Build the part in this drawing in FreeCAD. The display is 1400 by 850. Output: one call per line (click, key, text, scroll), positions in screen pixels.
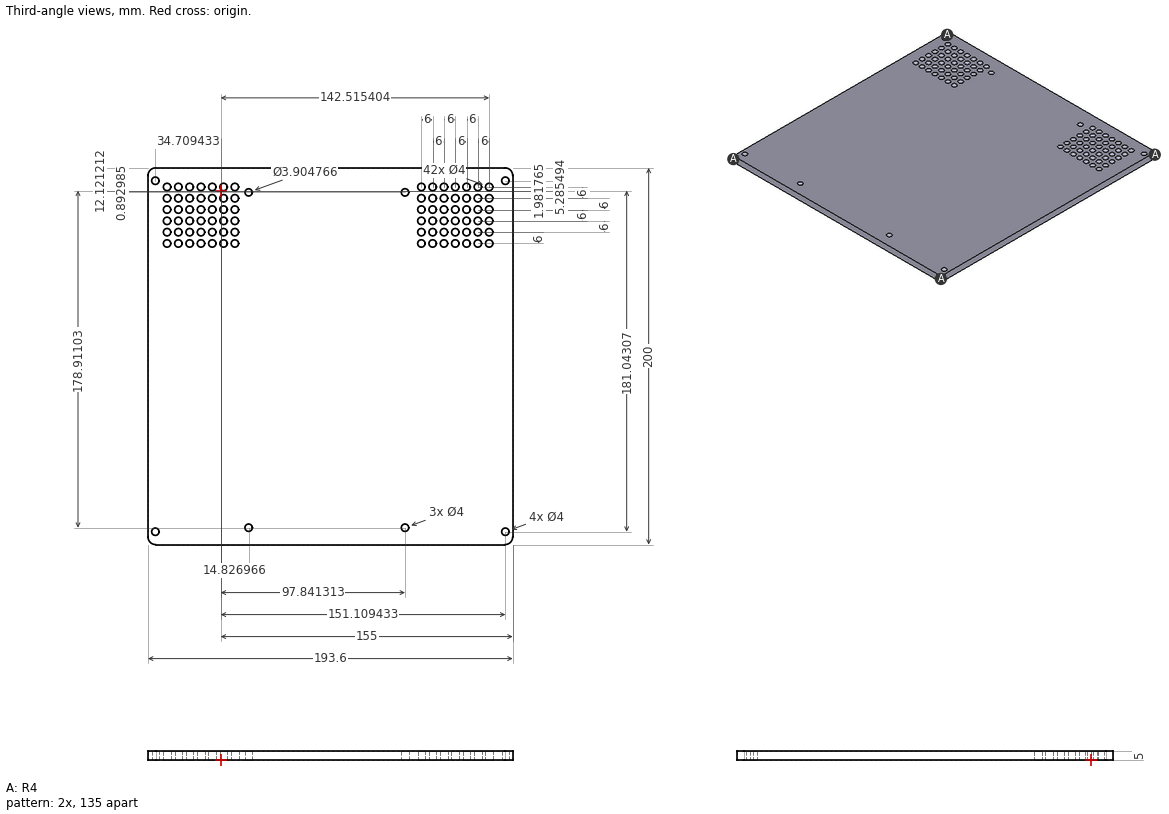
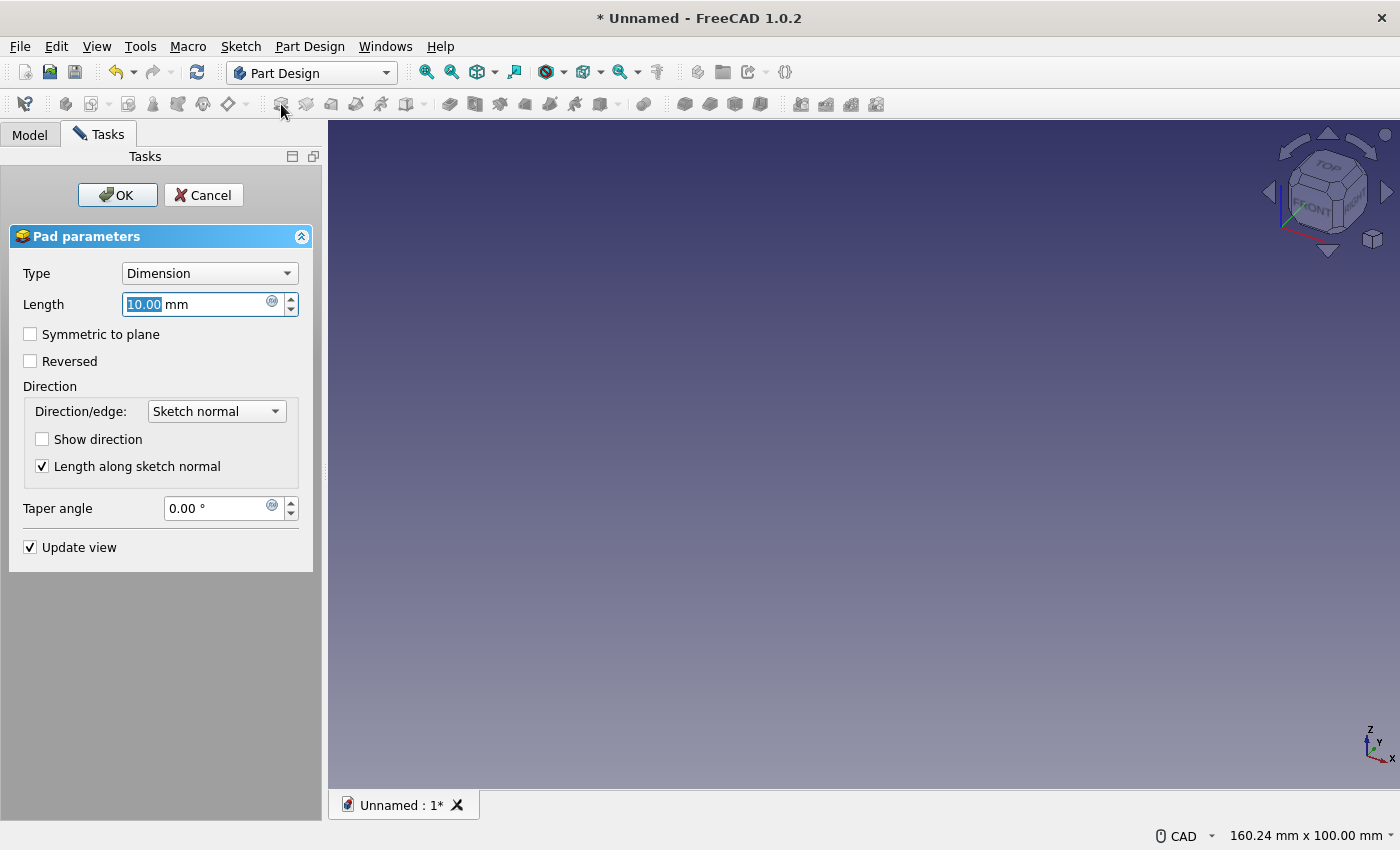
text(5)
key(Tab)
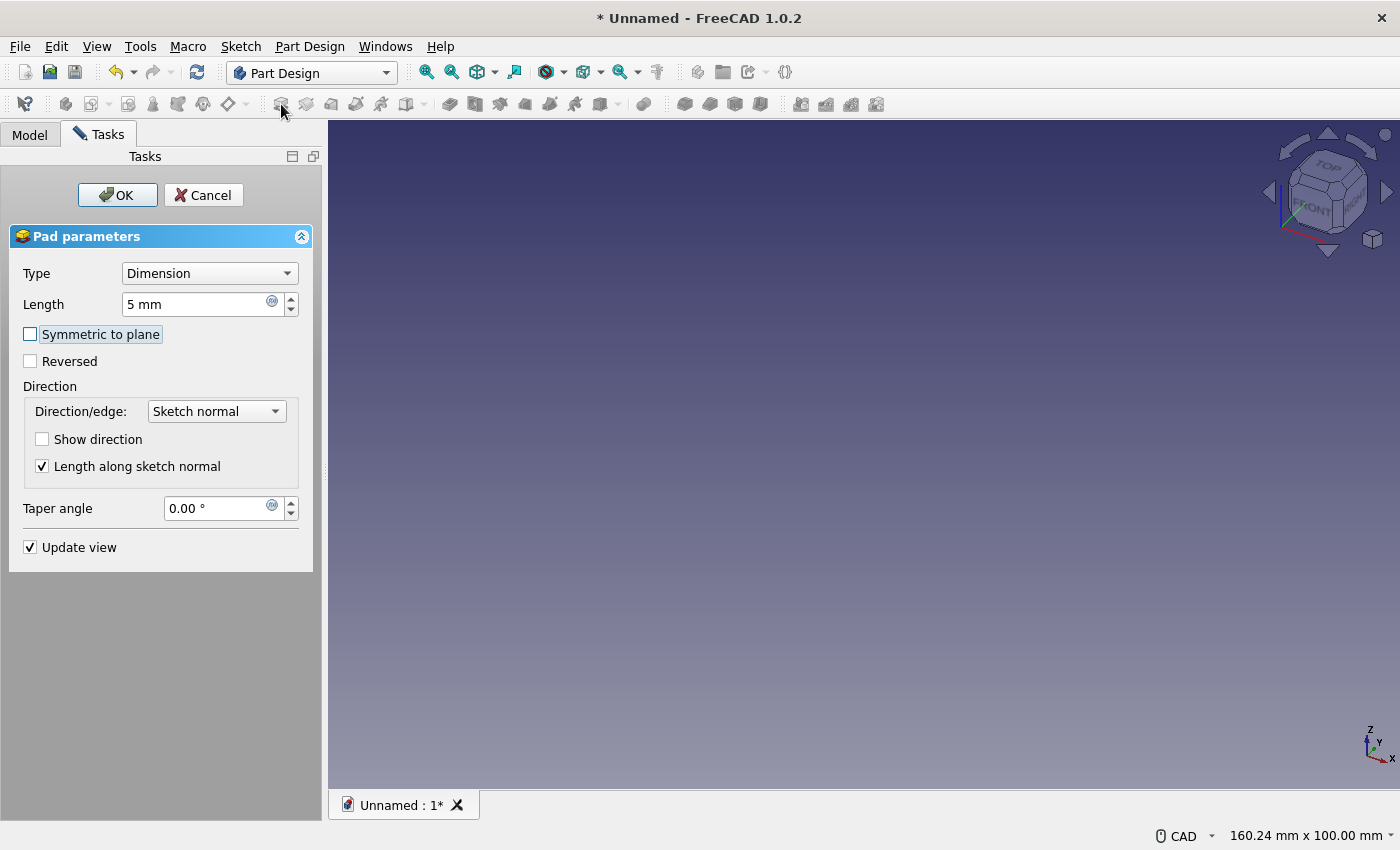
click(118, 195)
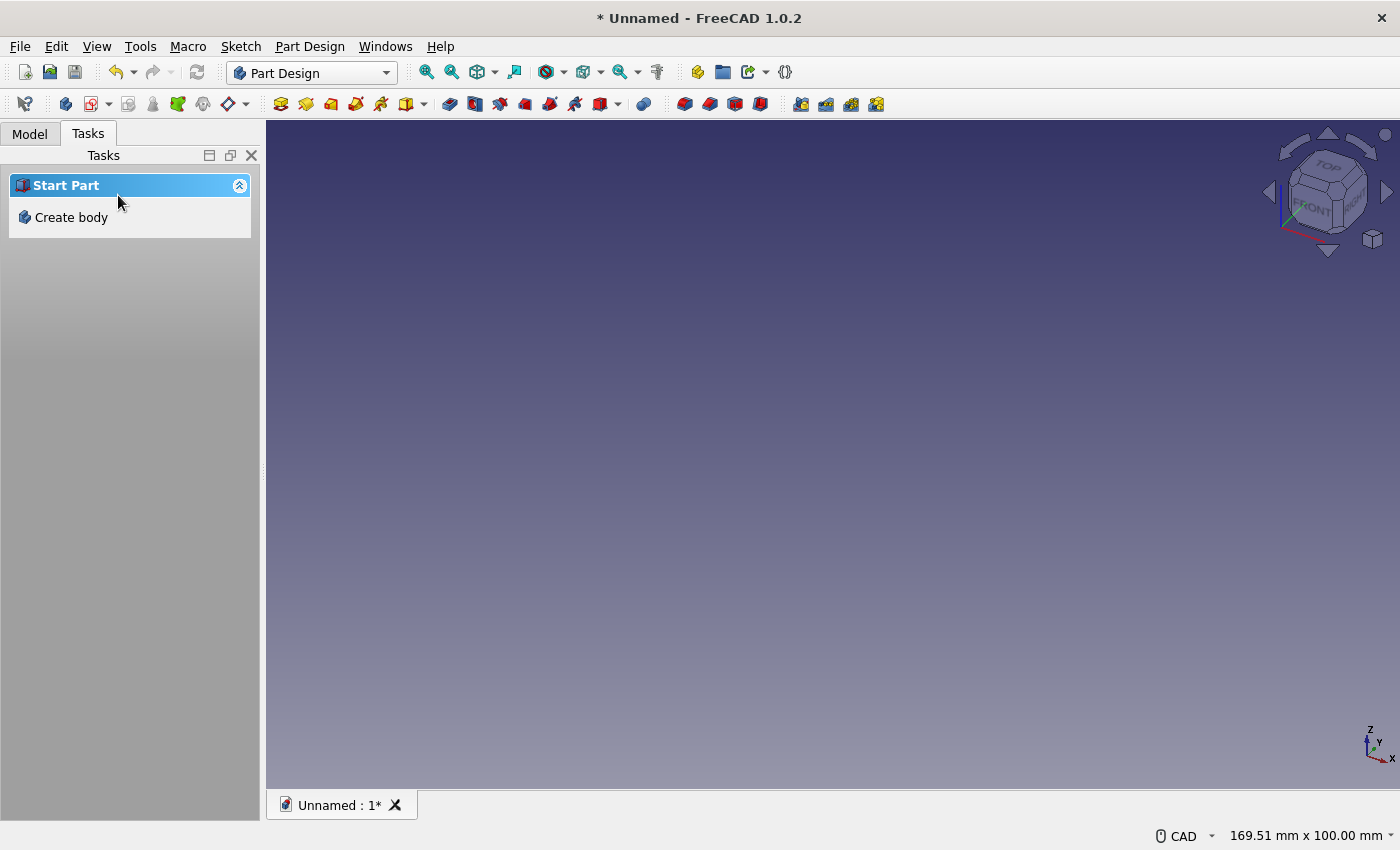
click(427, 72)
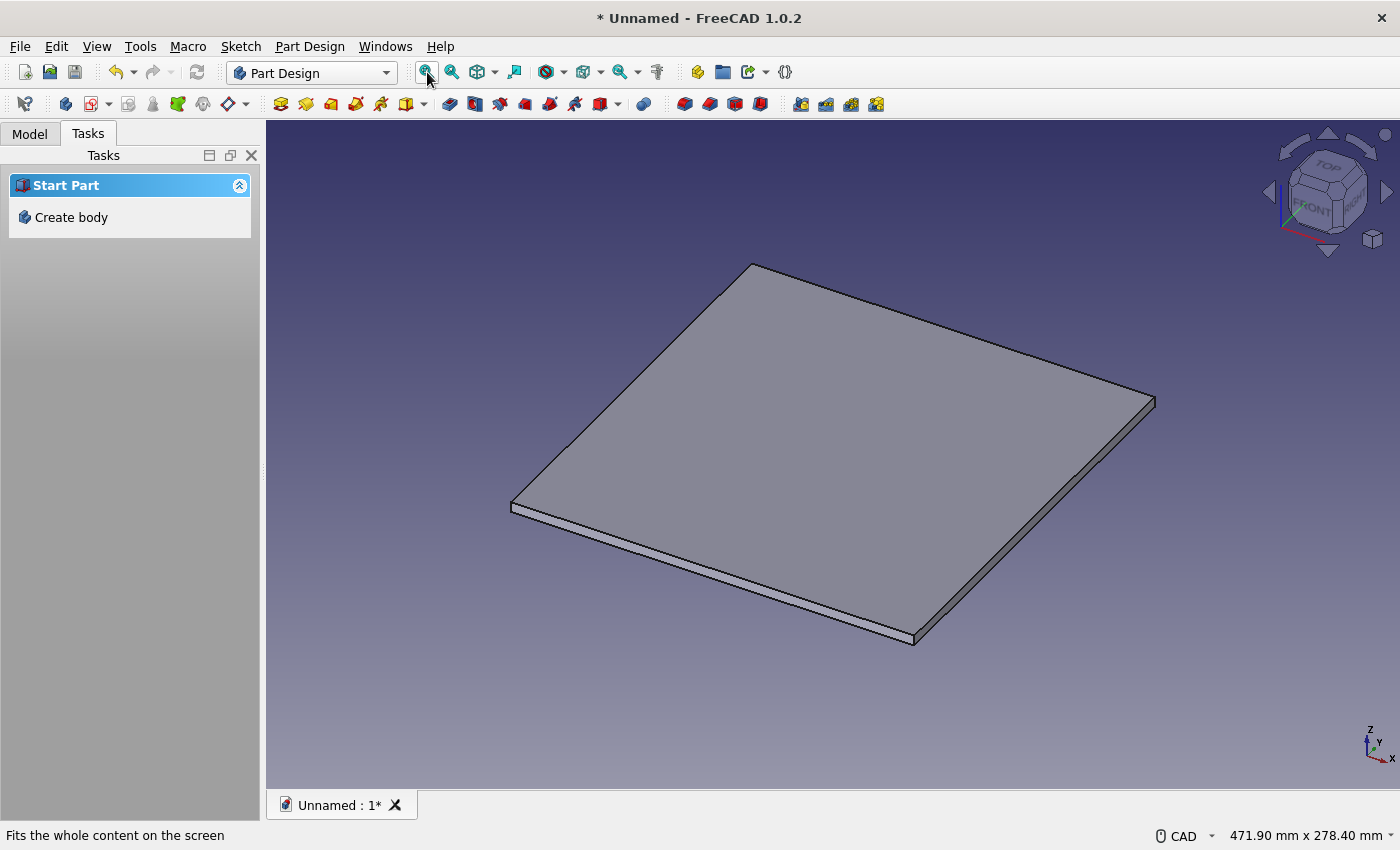
click(833, 449)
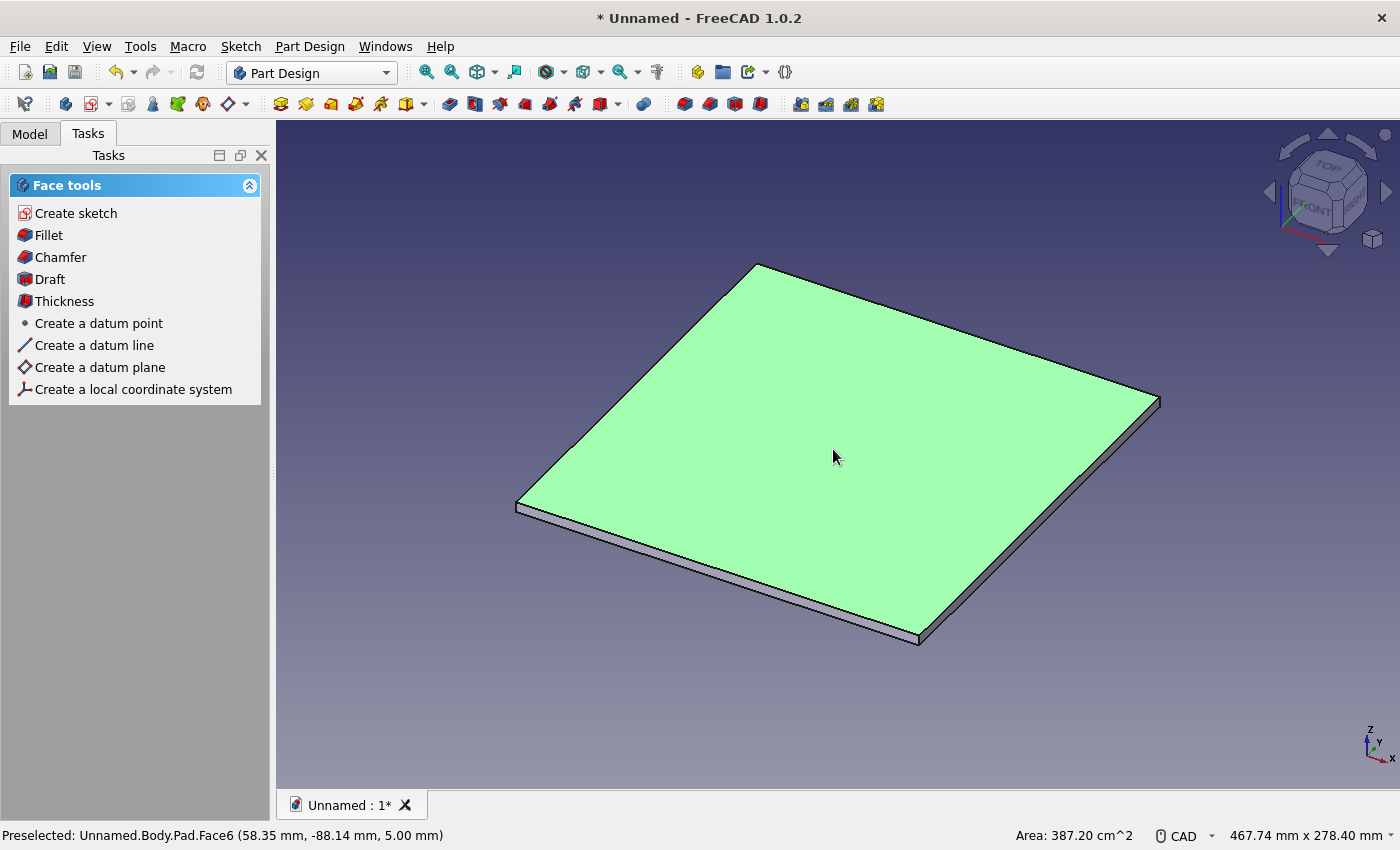
click(90, 104)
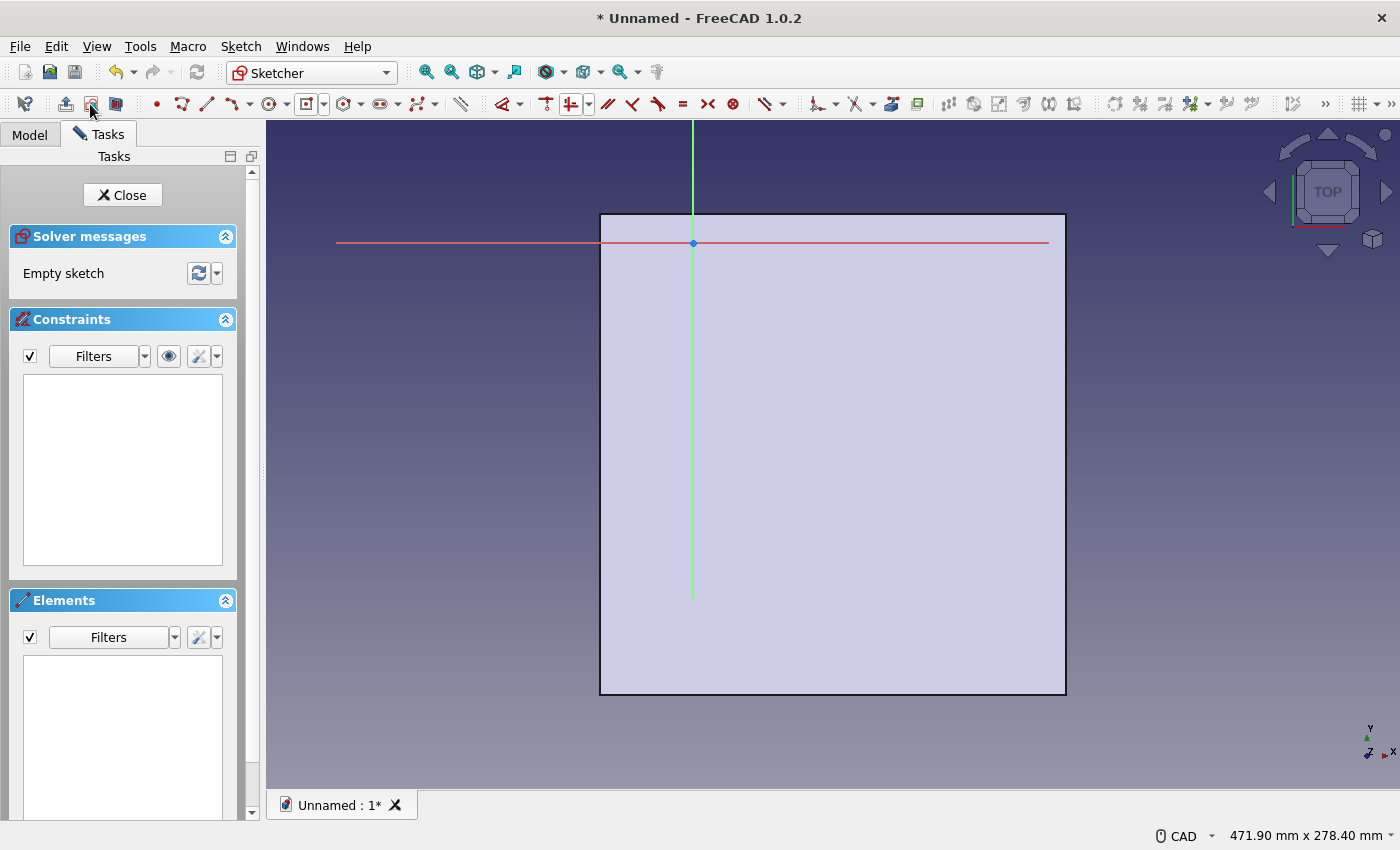
click(268, 104)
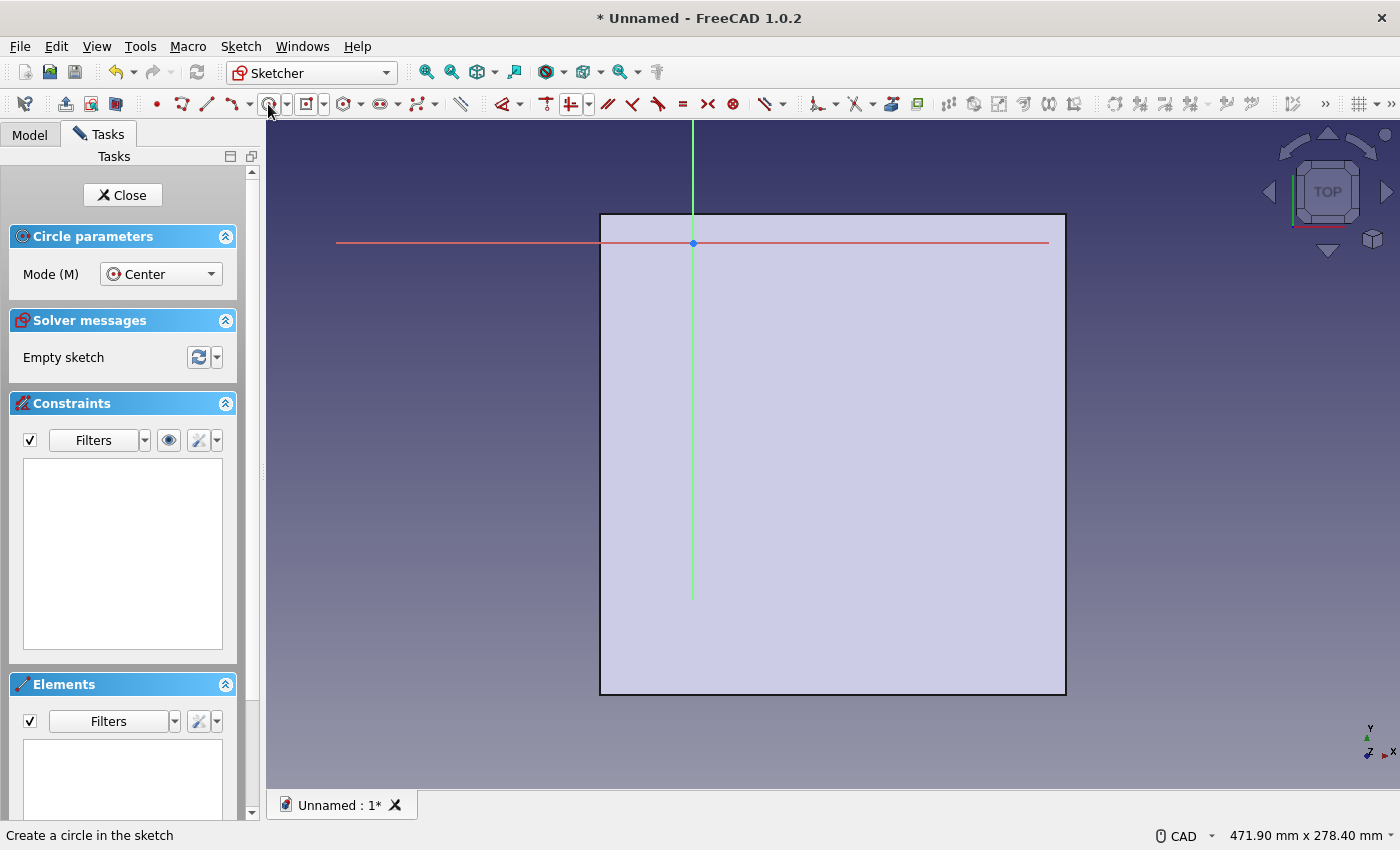
scroll(928, 673, up, 8)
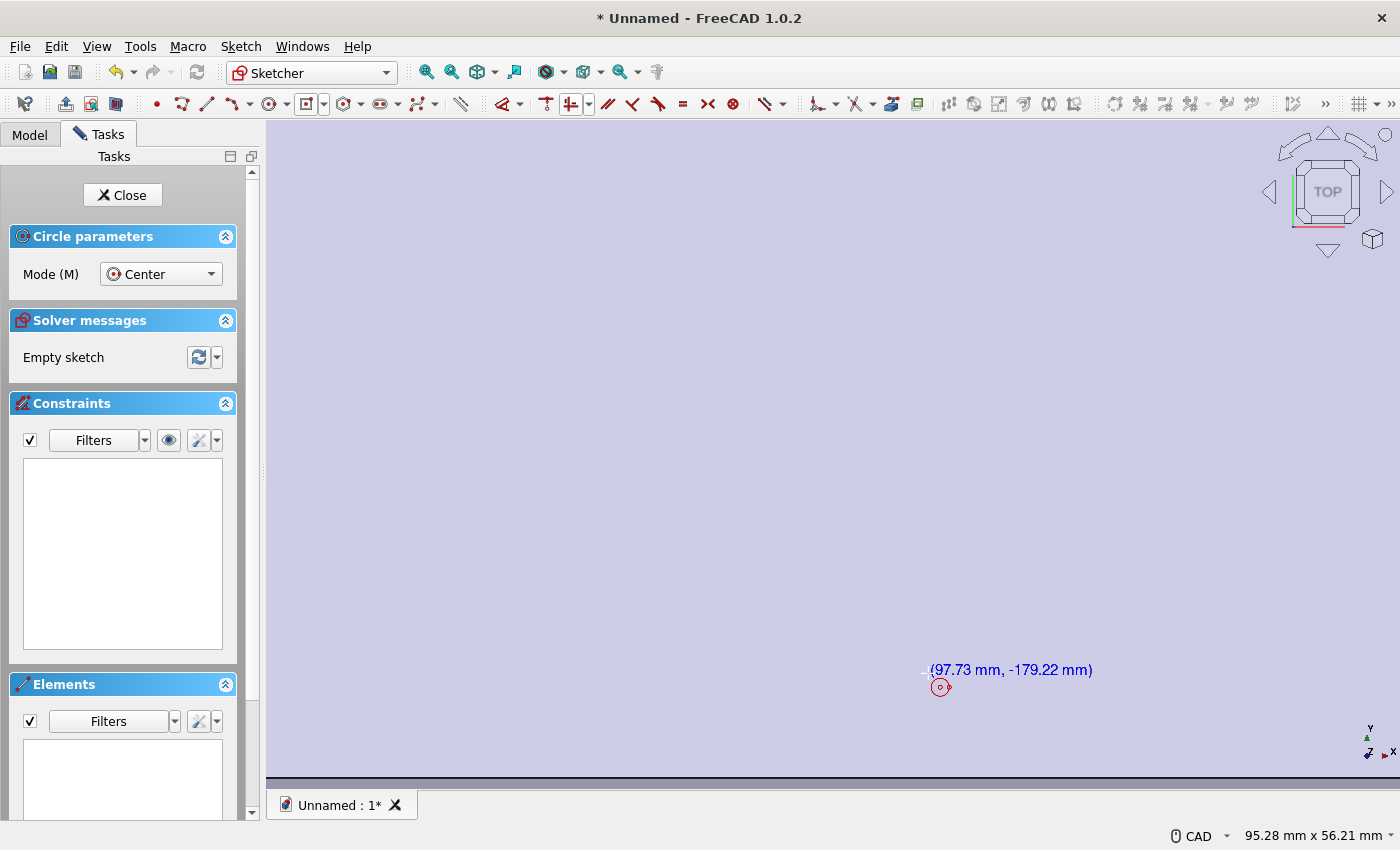
scroll(868, 668, down, 8)